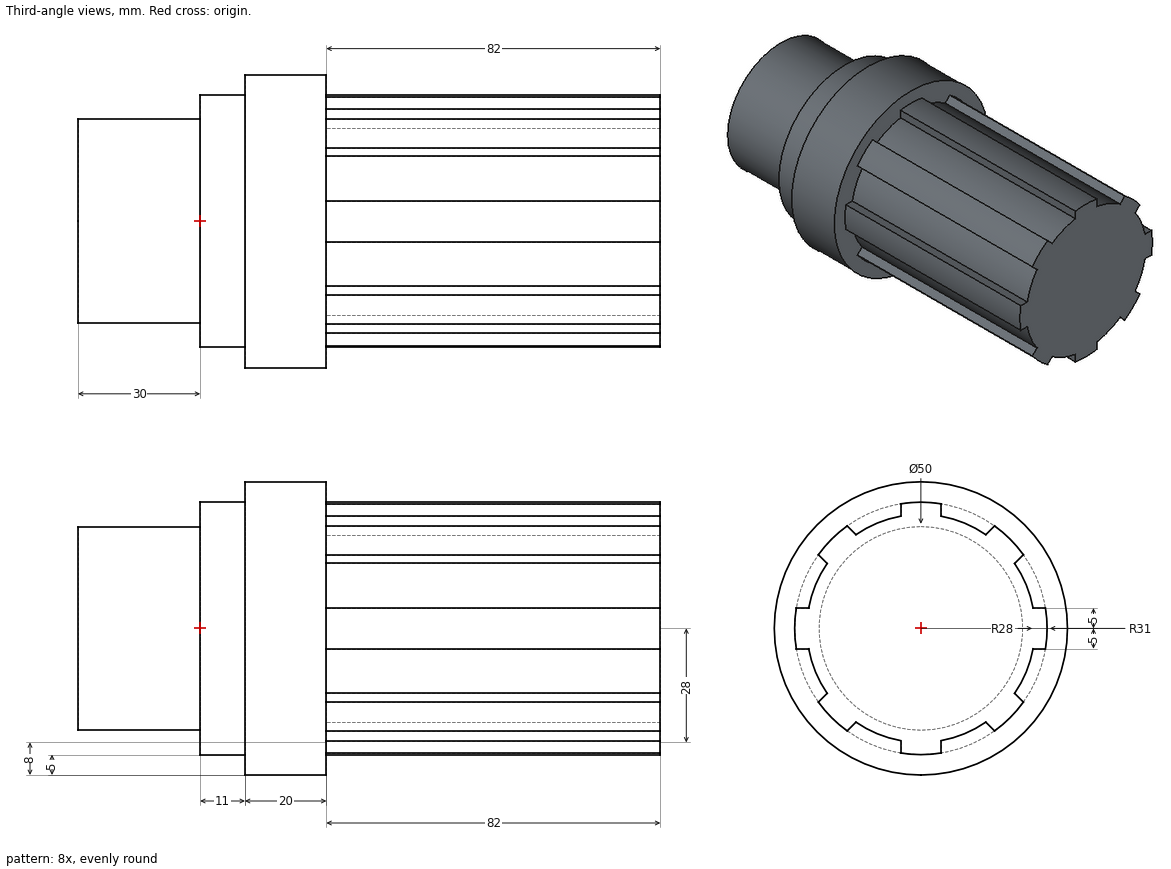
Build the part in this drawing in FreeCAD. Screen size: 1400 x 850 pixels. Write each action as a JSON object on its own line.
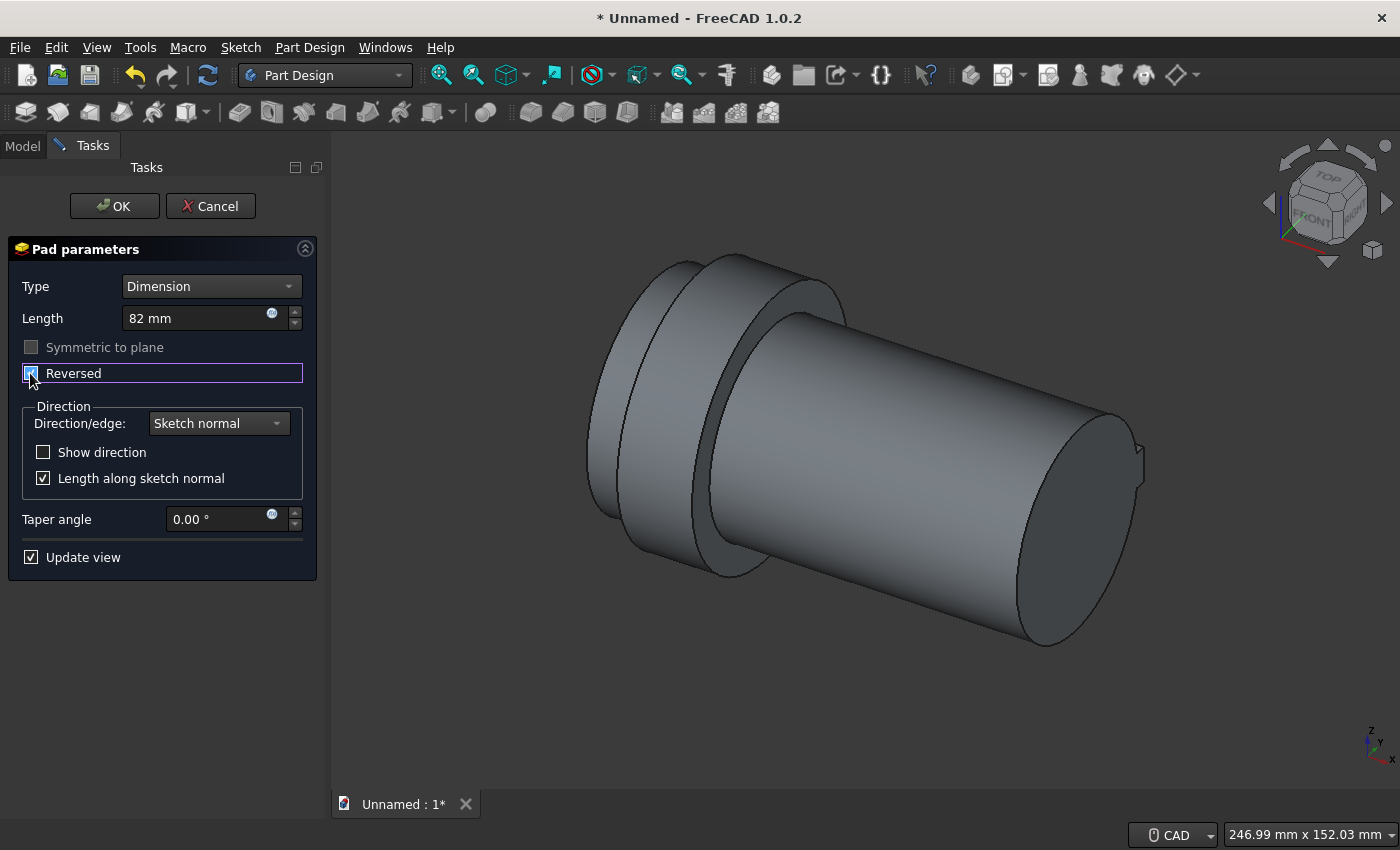
{"action": "left_click", "coordinate": [115, 206]}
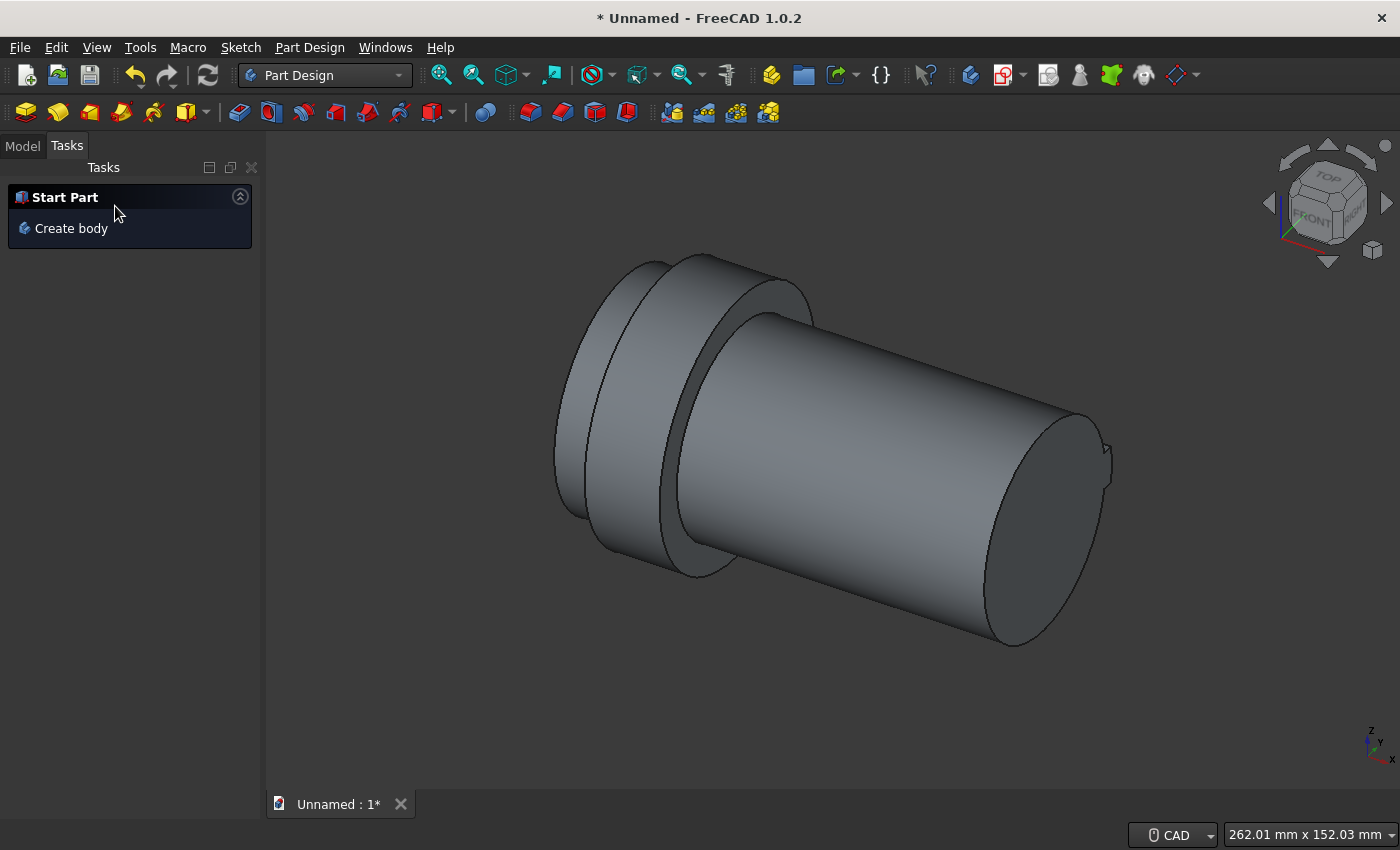
{"action": "left_click", "coordinate": [23, 145]}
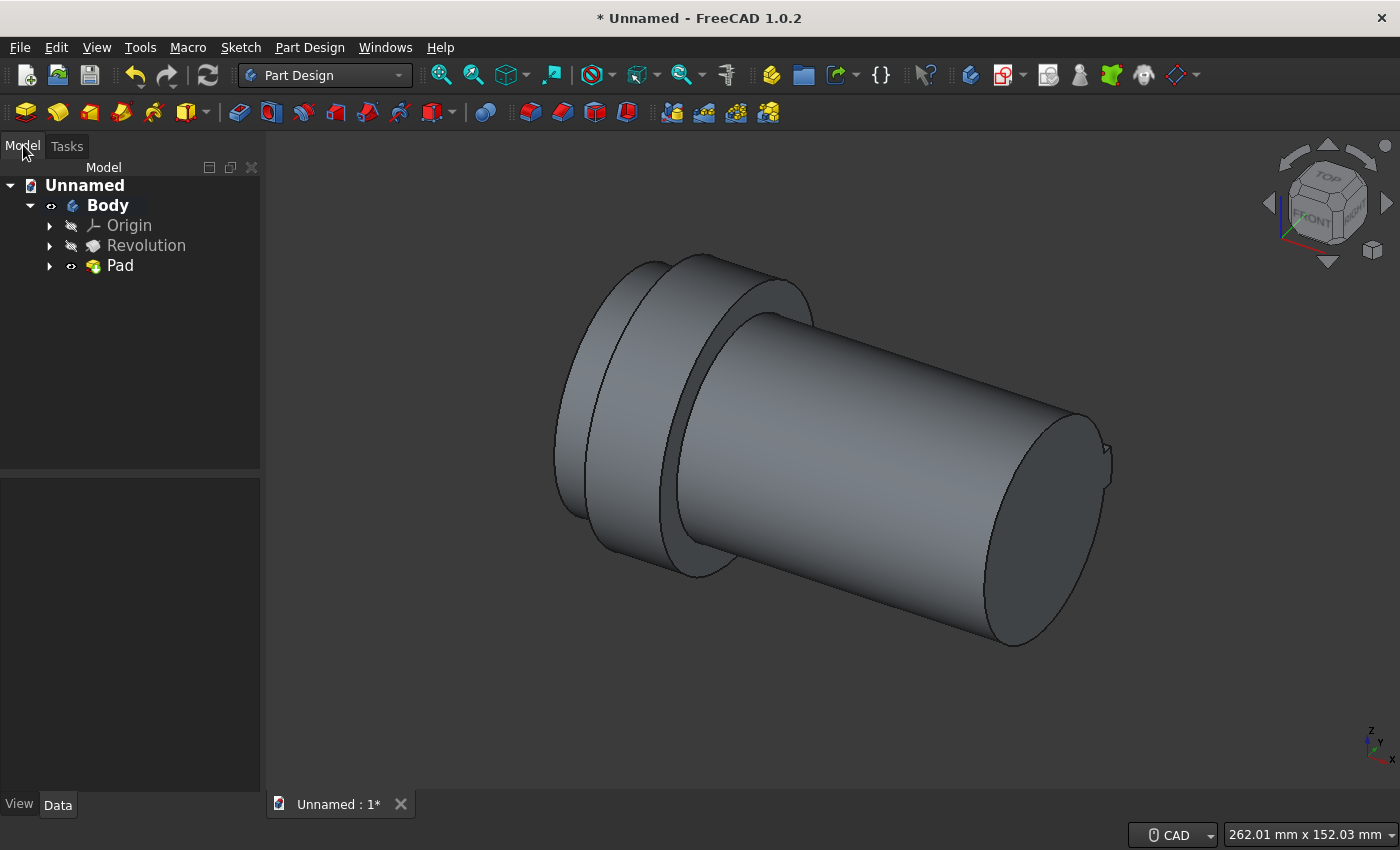
{"action": "left_click", "coordinate": [116, 266]}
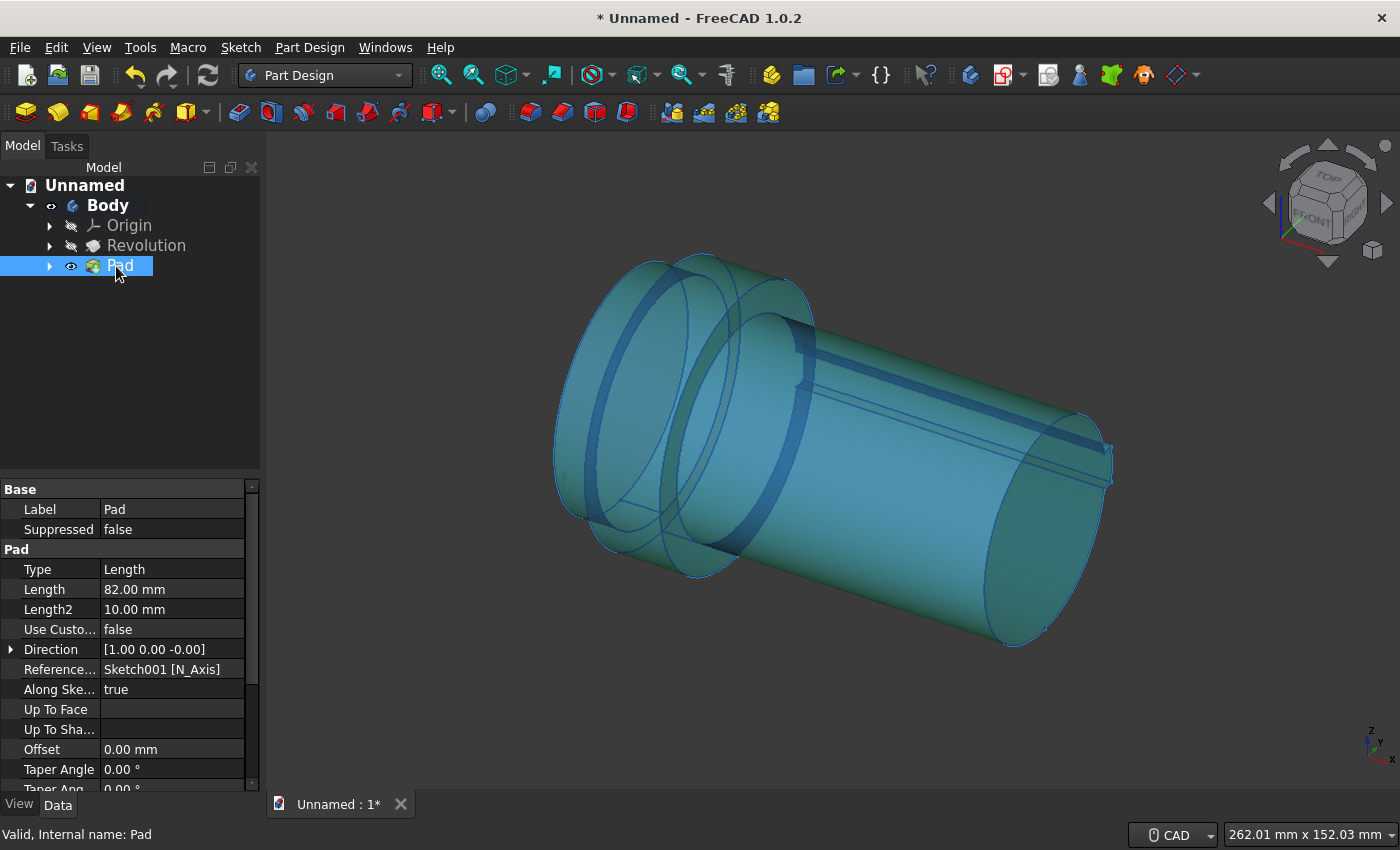
{"action": "left_click", "coordinate": [736, 112]}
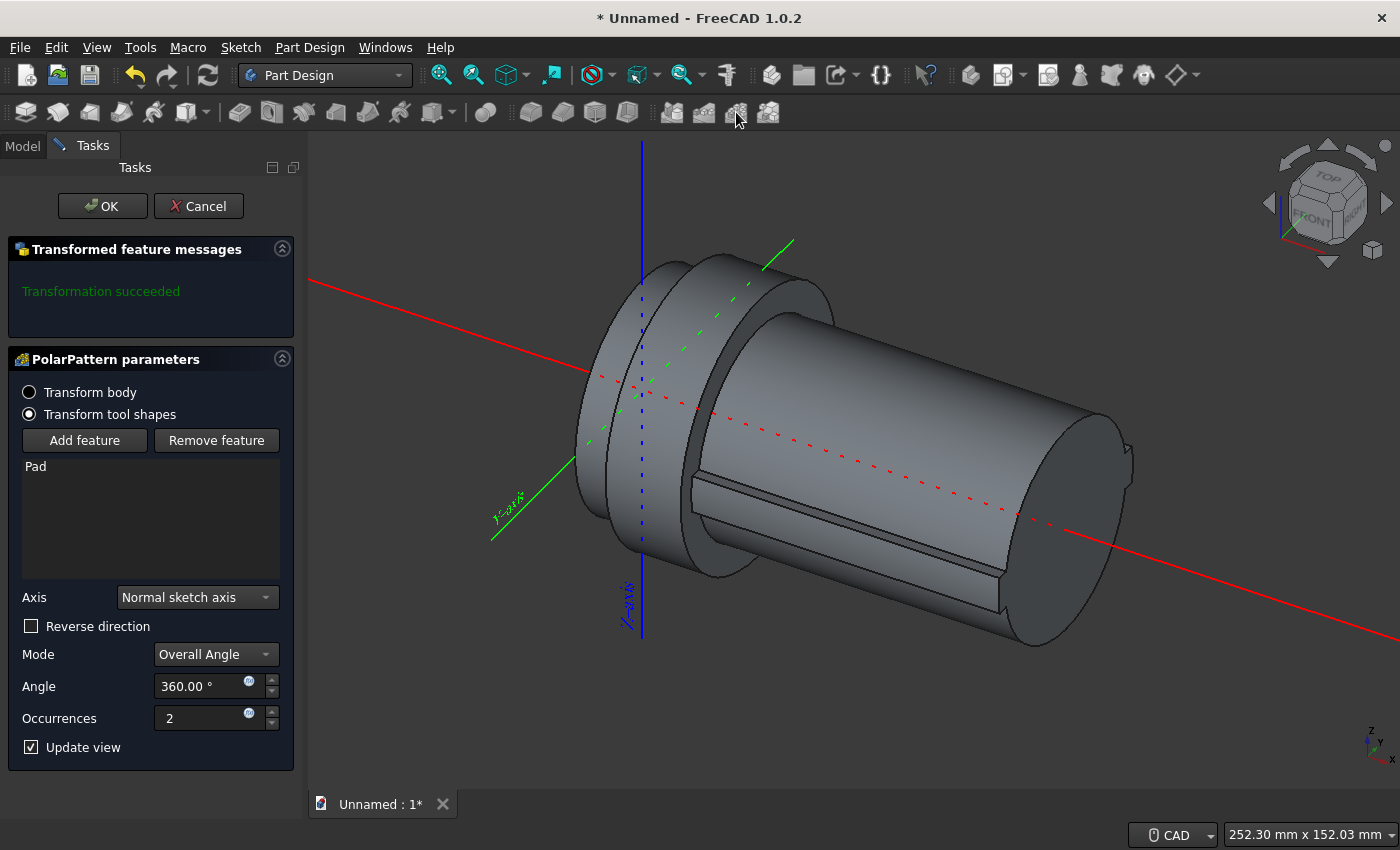
{"action": "left_click", "coordinate": [198, 598]}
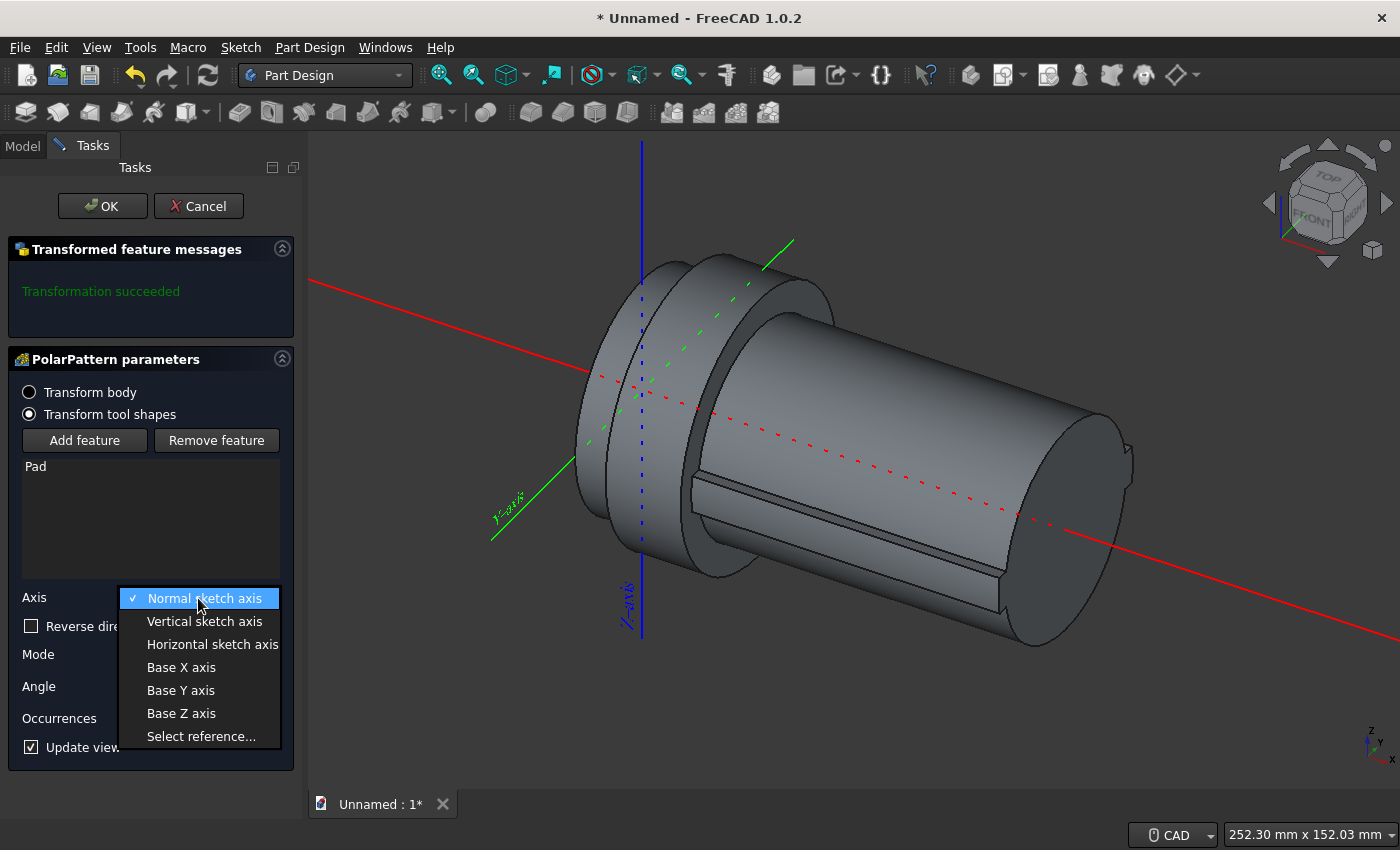
{"action": "left_click", "coordinate": [198, 668]}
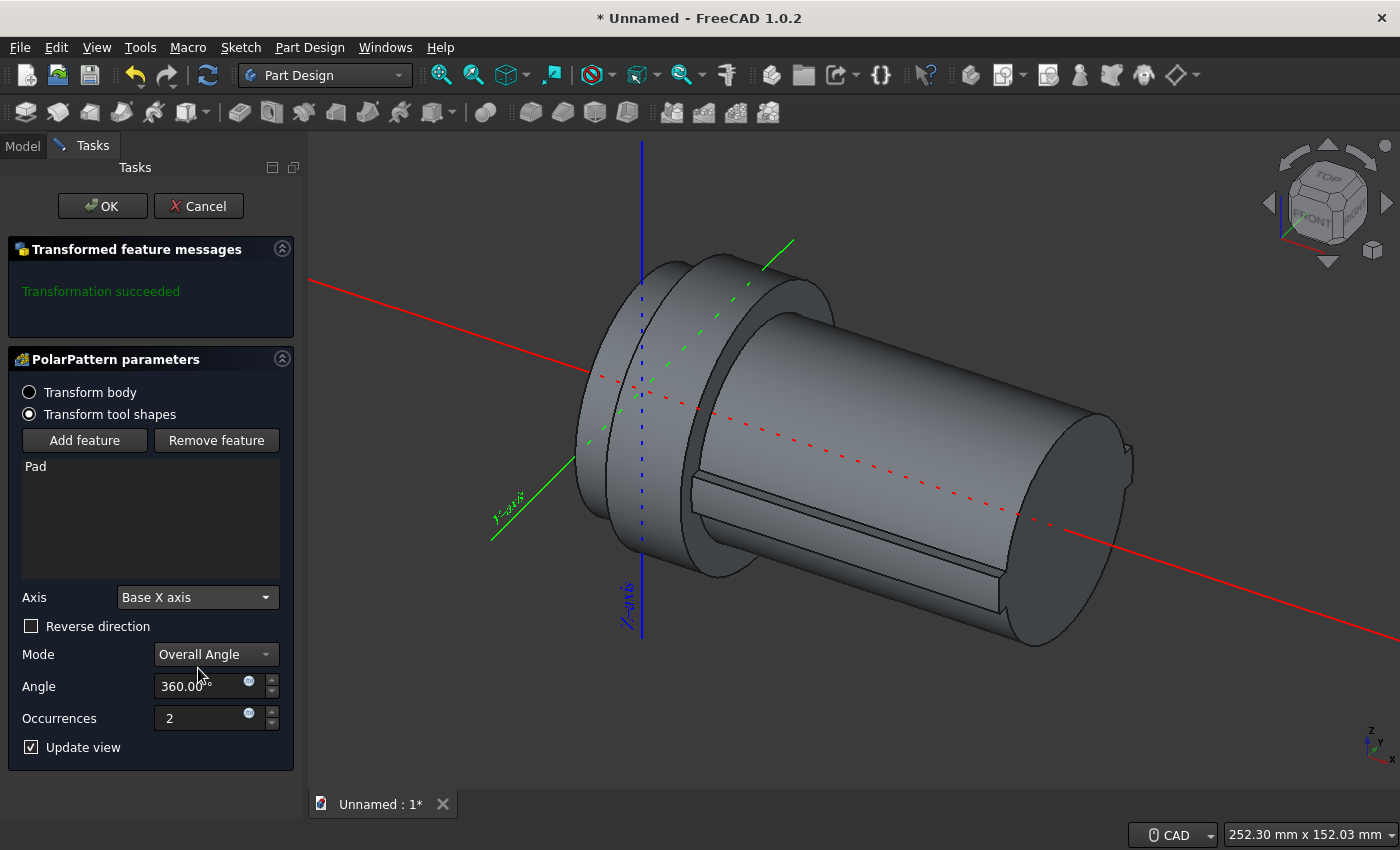
{"action": "triple_click", "coordinate": [209, 718]}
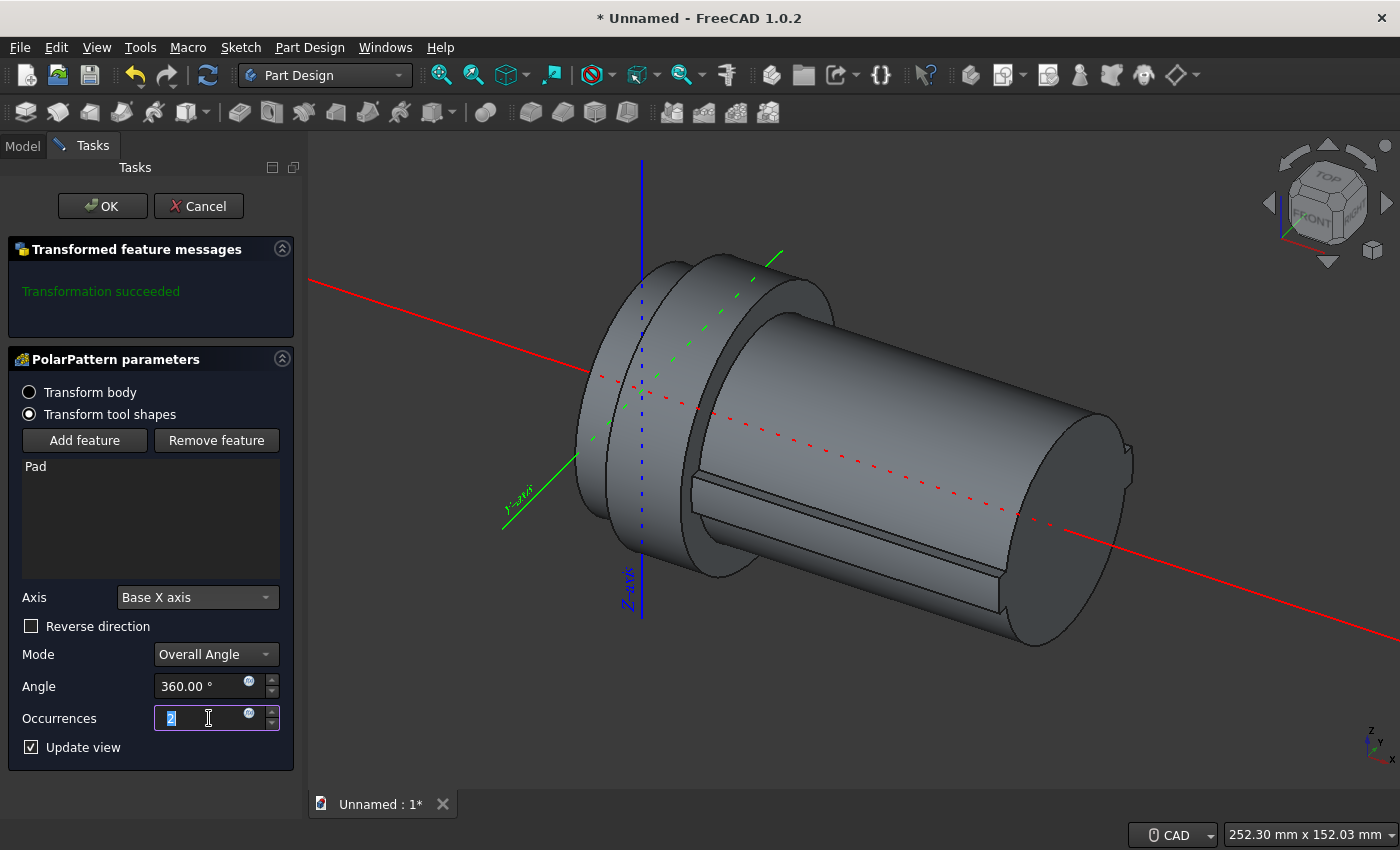
{"action": "type", "text": "8"}
{"action": "key", "text": "Tab"}